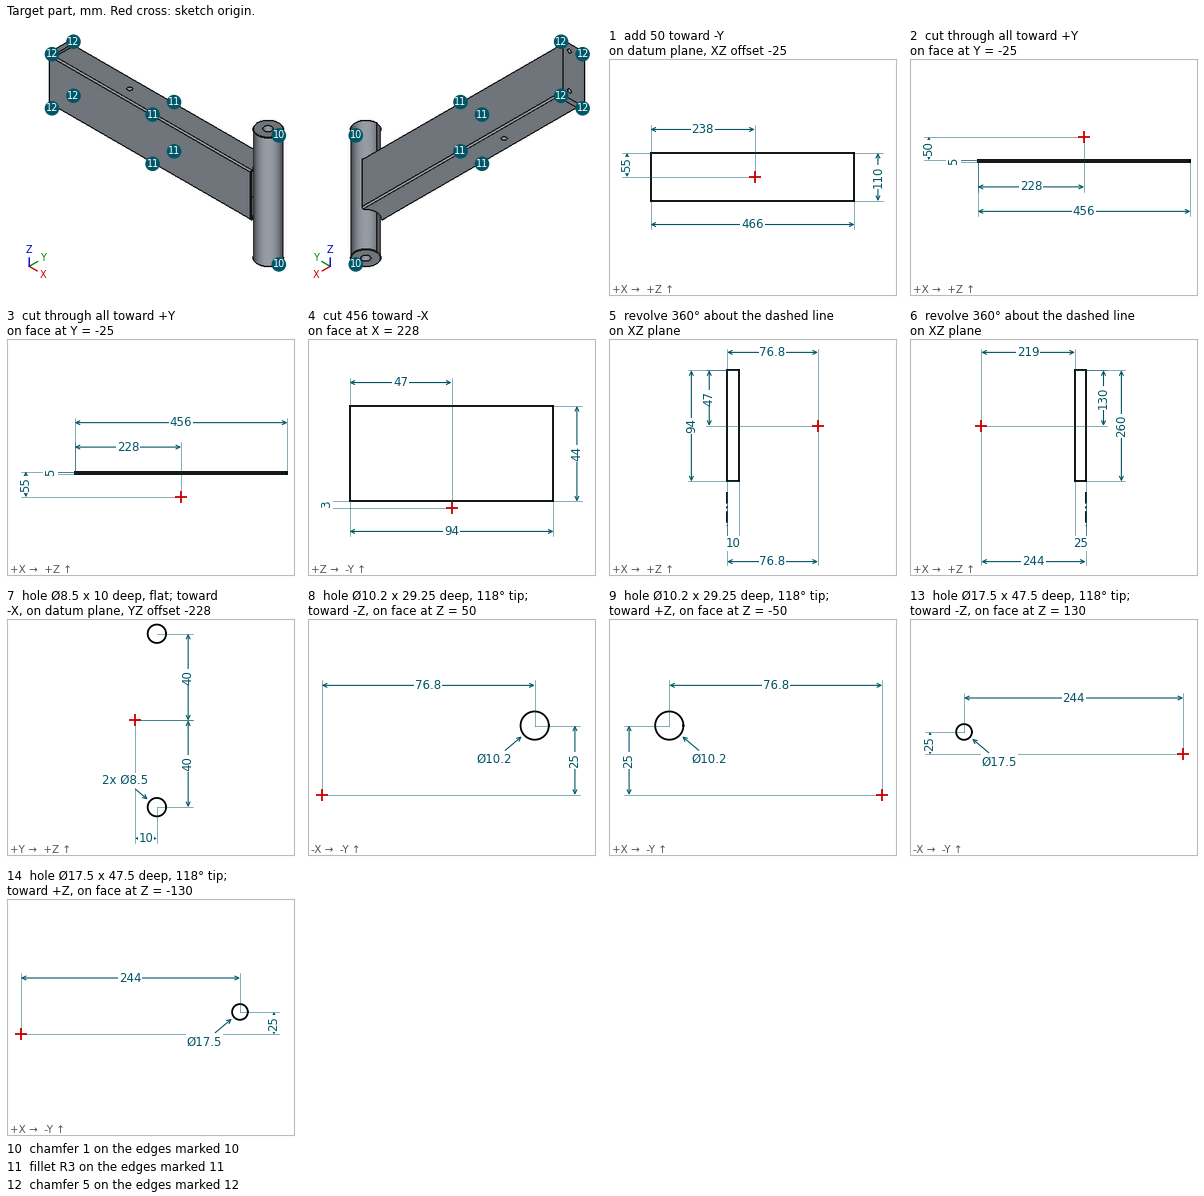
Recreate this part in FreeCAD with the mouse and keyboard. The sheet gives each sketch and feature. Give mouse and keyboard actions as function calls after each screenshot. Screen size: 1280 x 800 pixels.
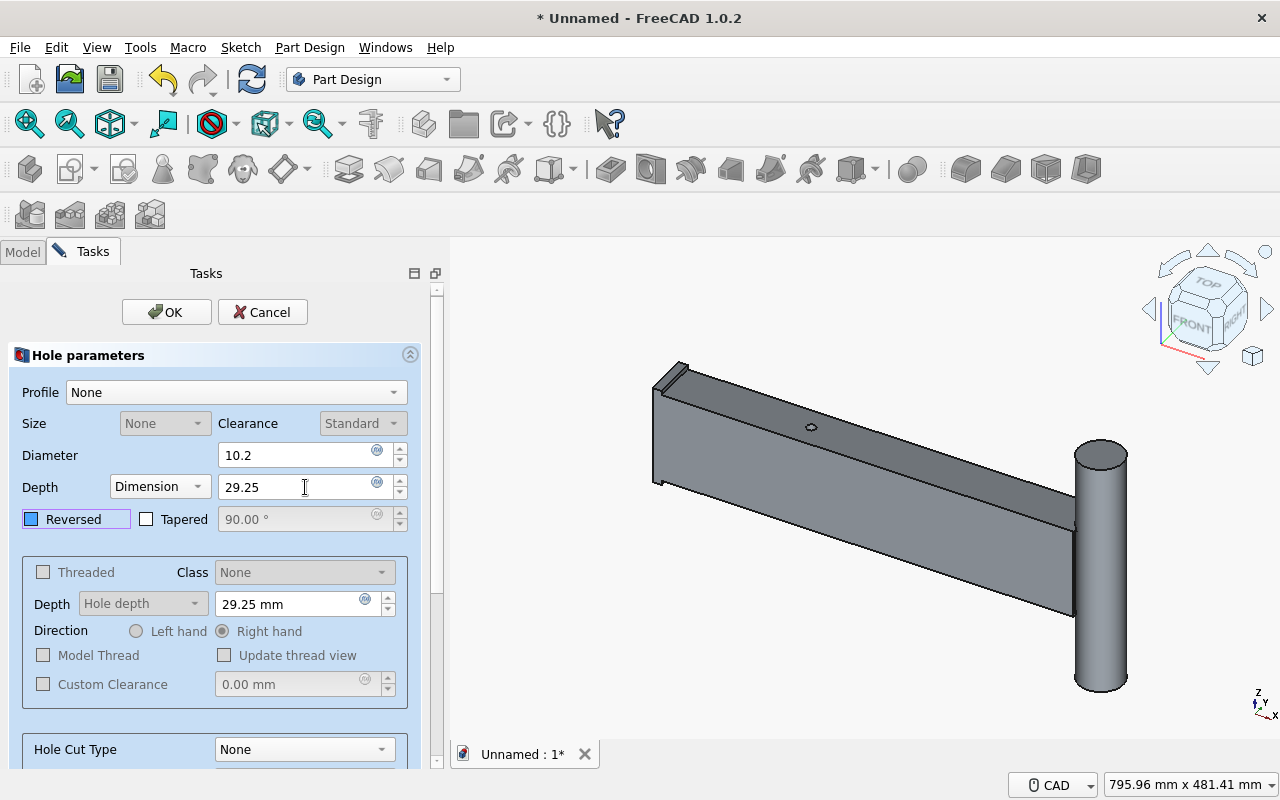
click(167, 312)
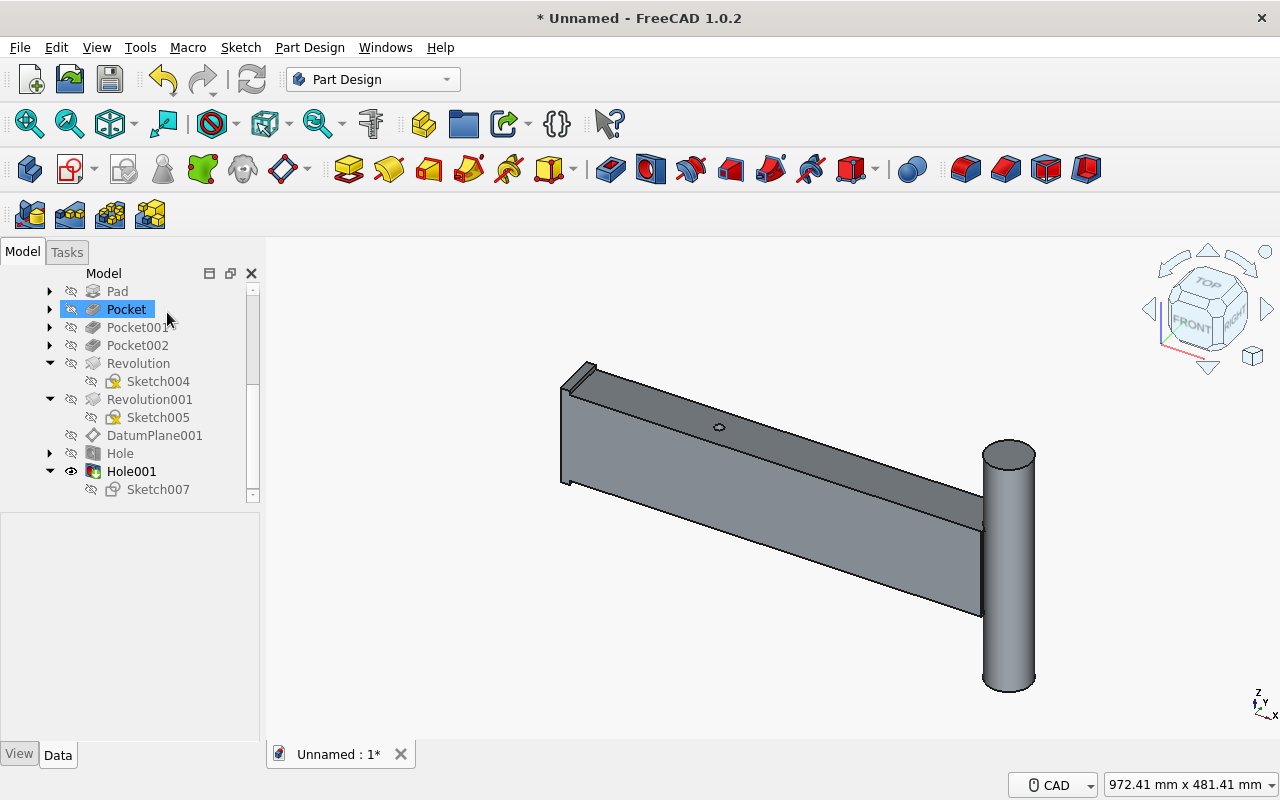
key(5)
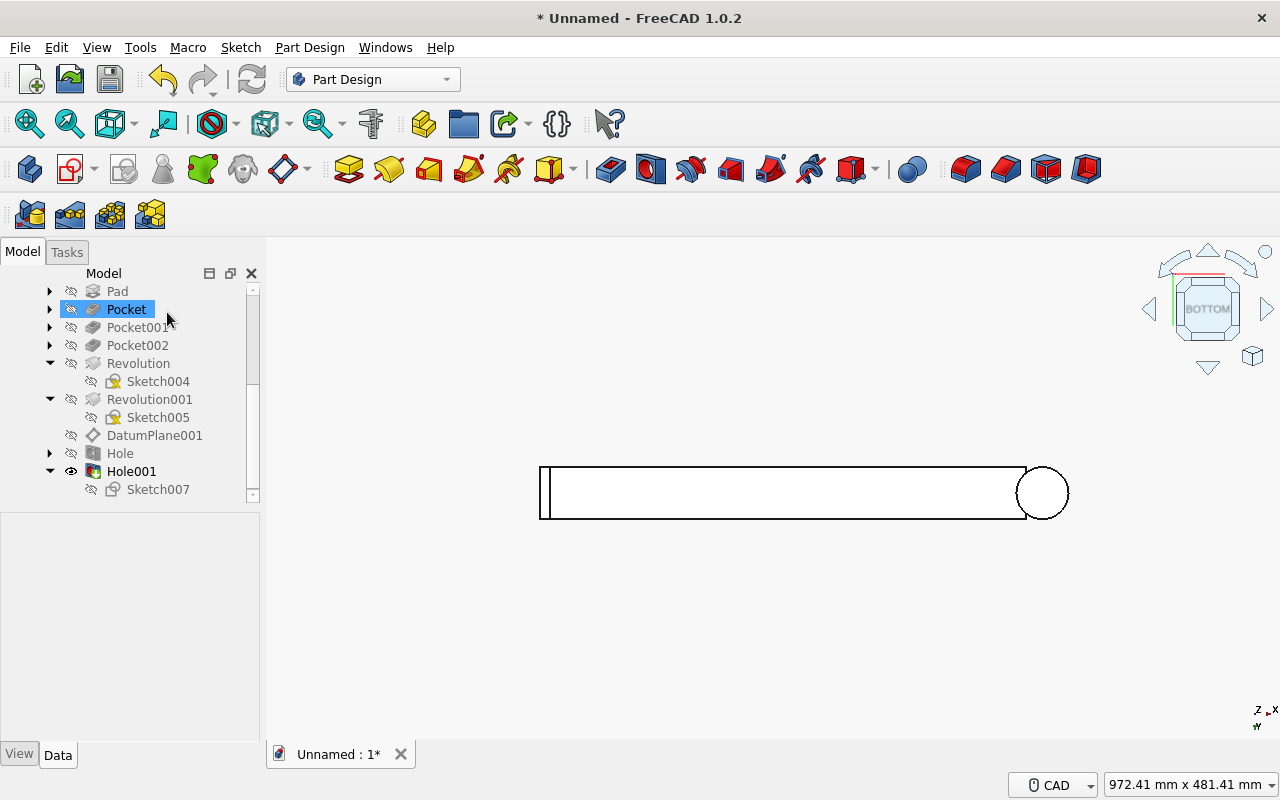
click(924, 492)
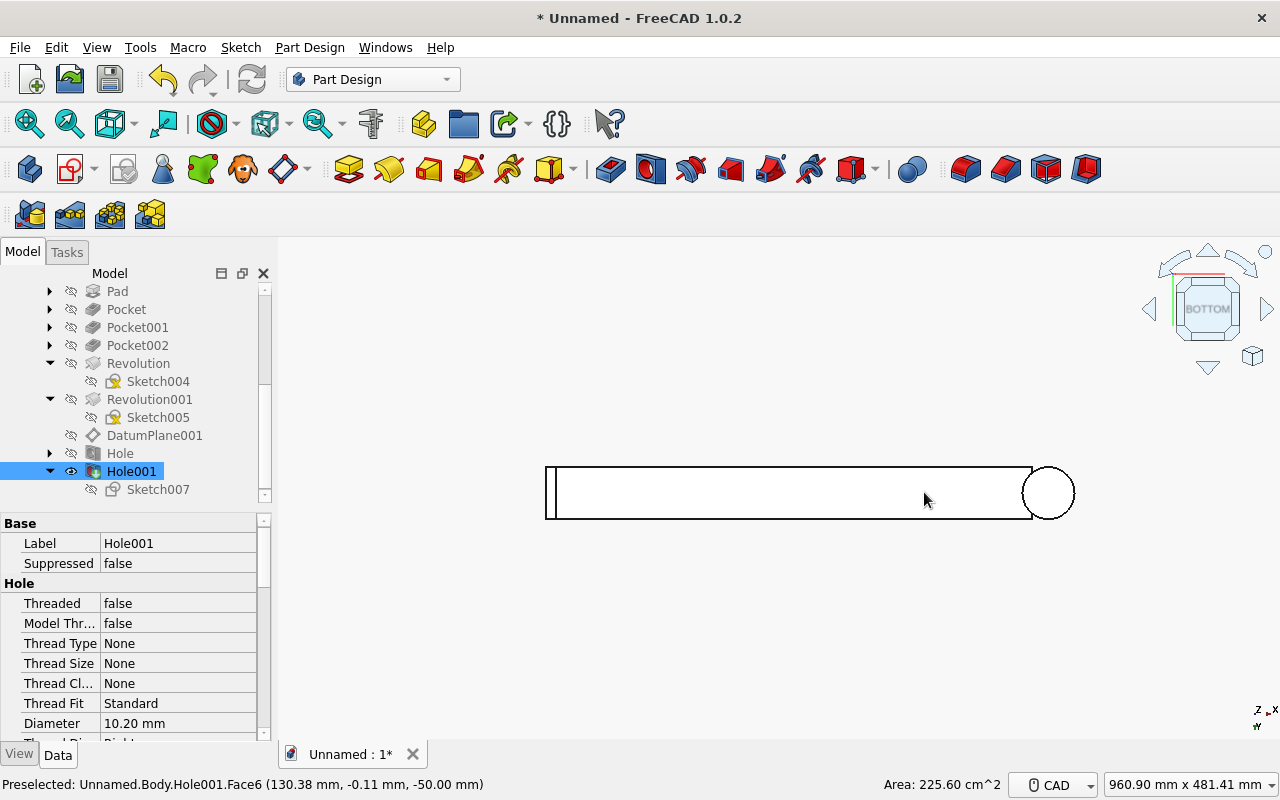
click(70, 170)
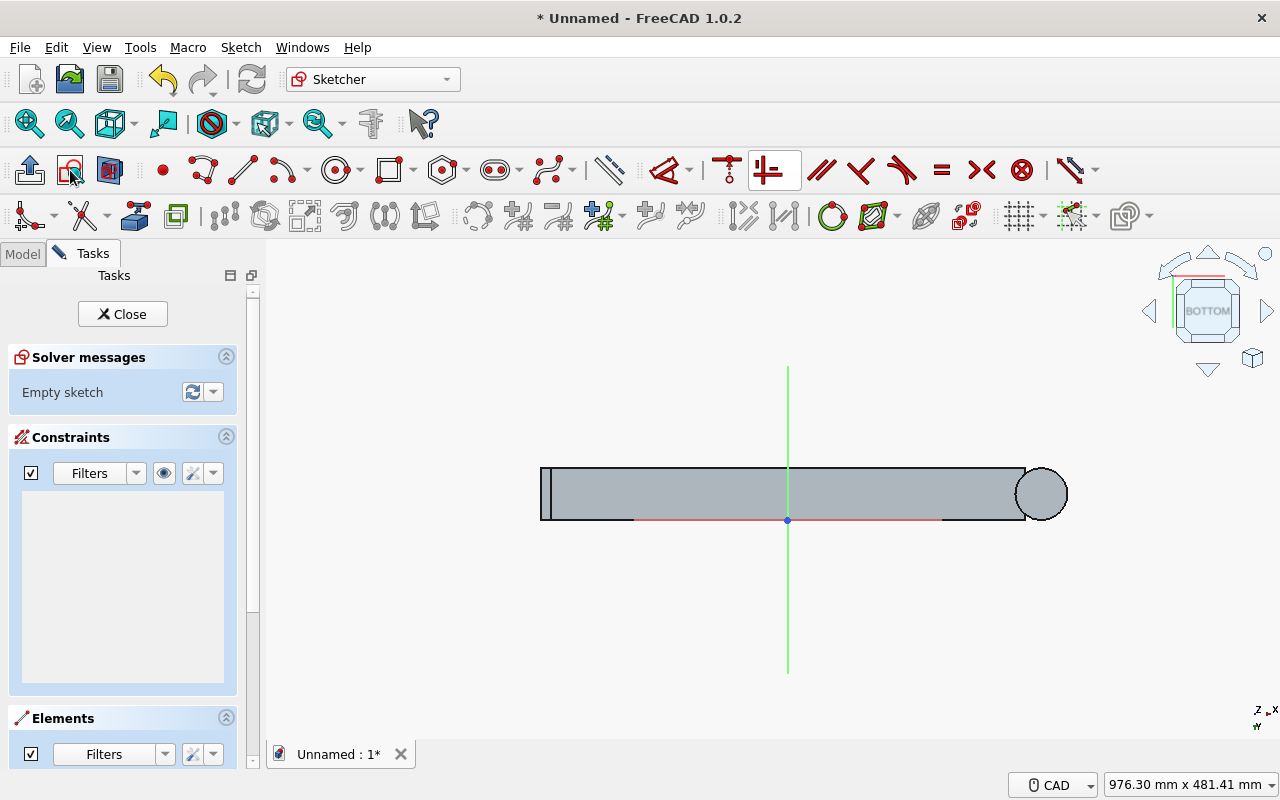
click(110, 170)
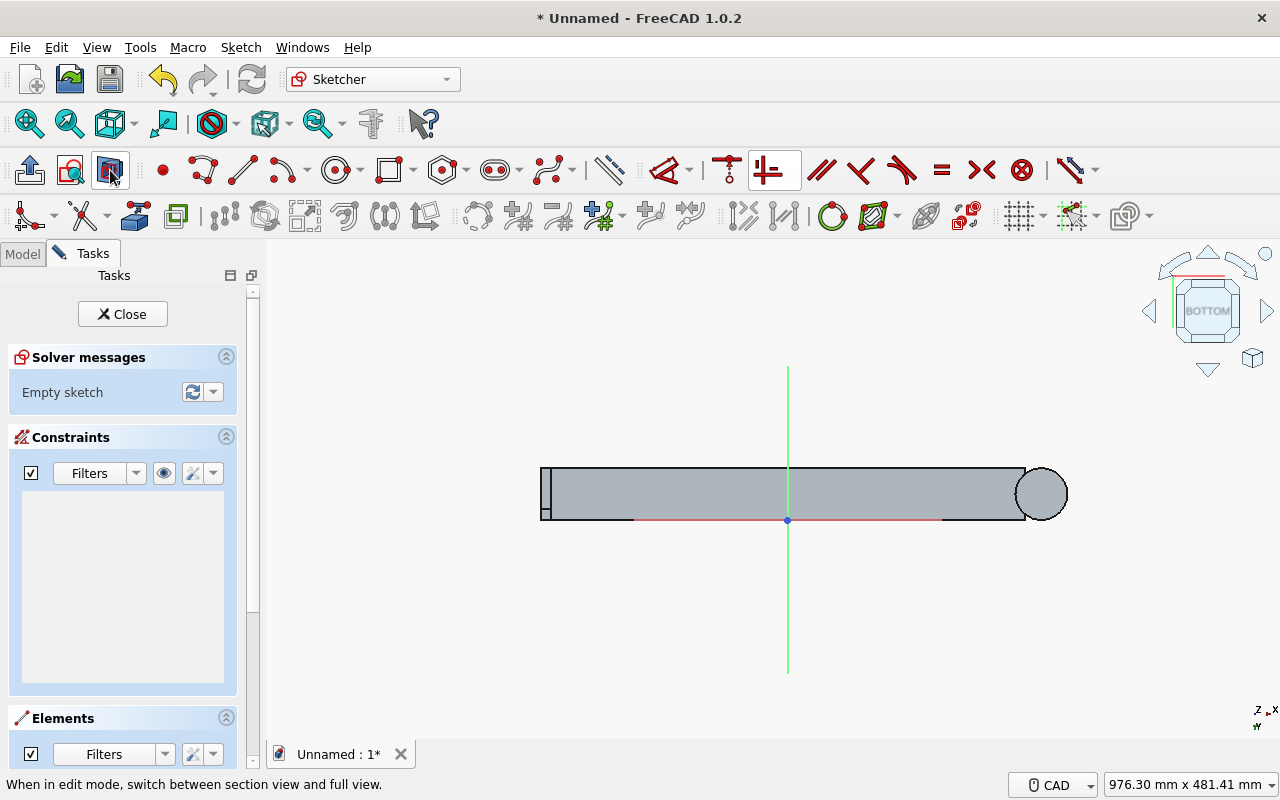
scroll(708, 494, up, 15)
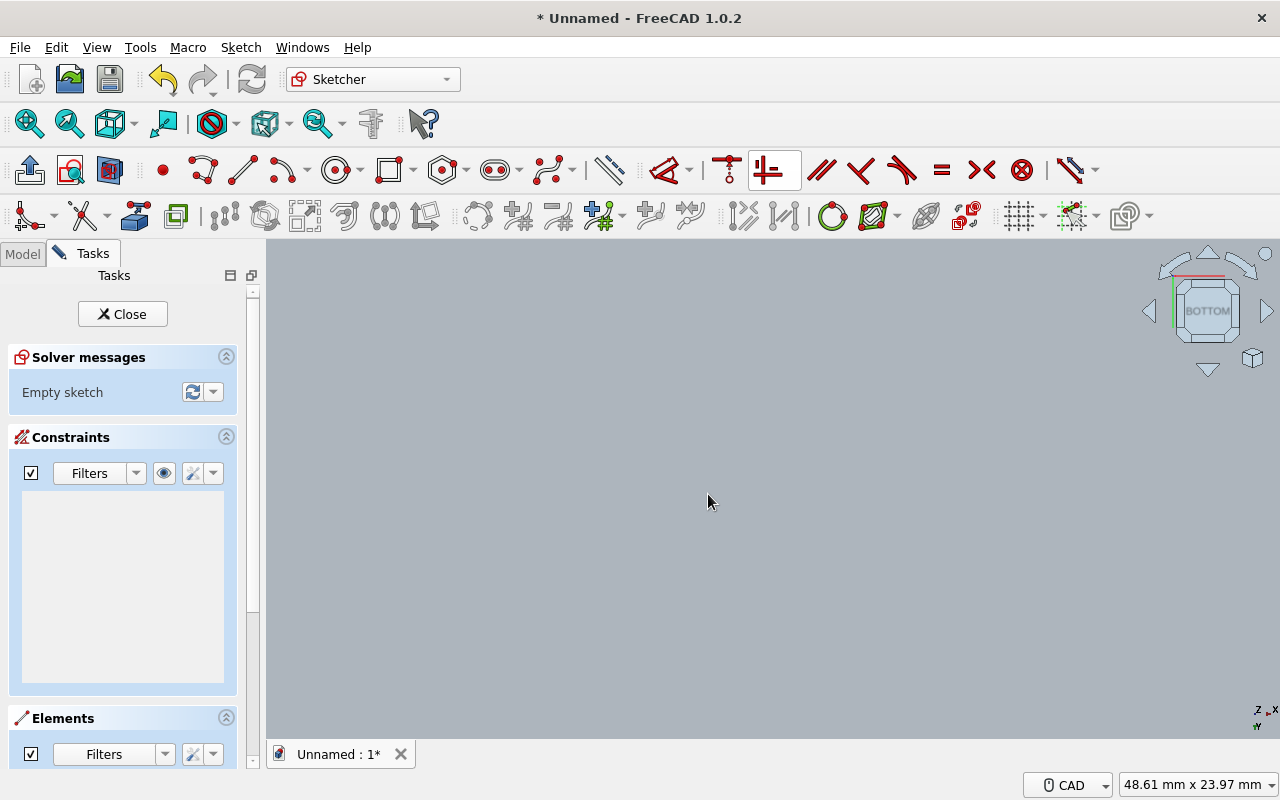
scroll(703, 481, up, 2)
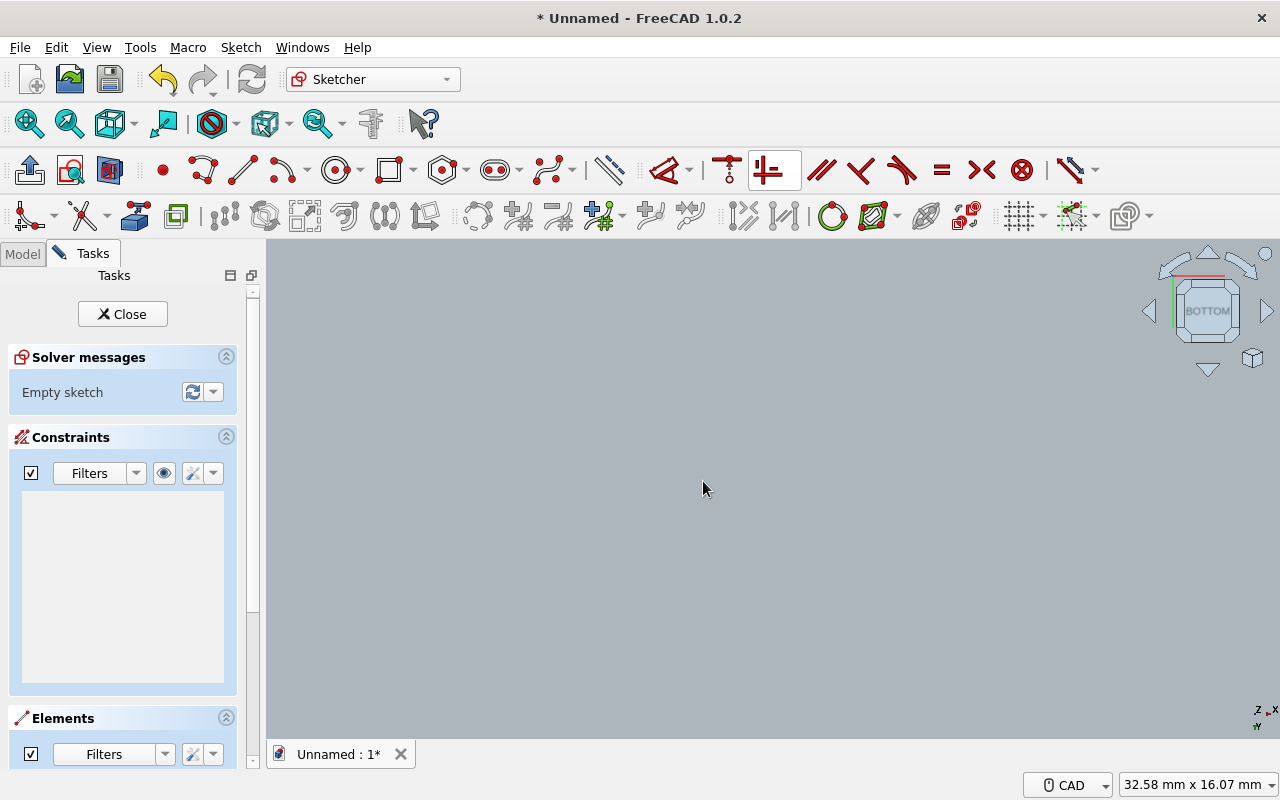
click(336, 170)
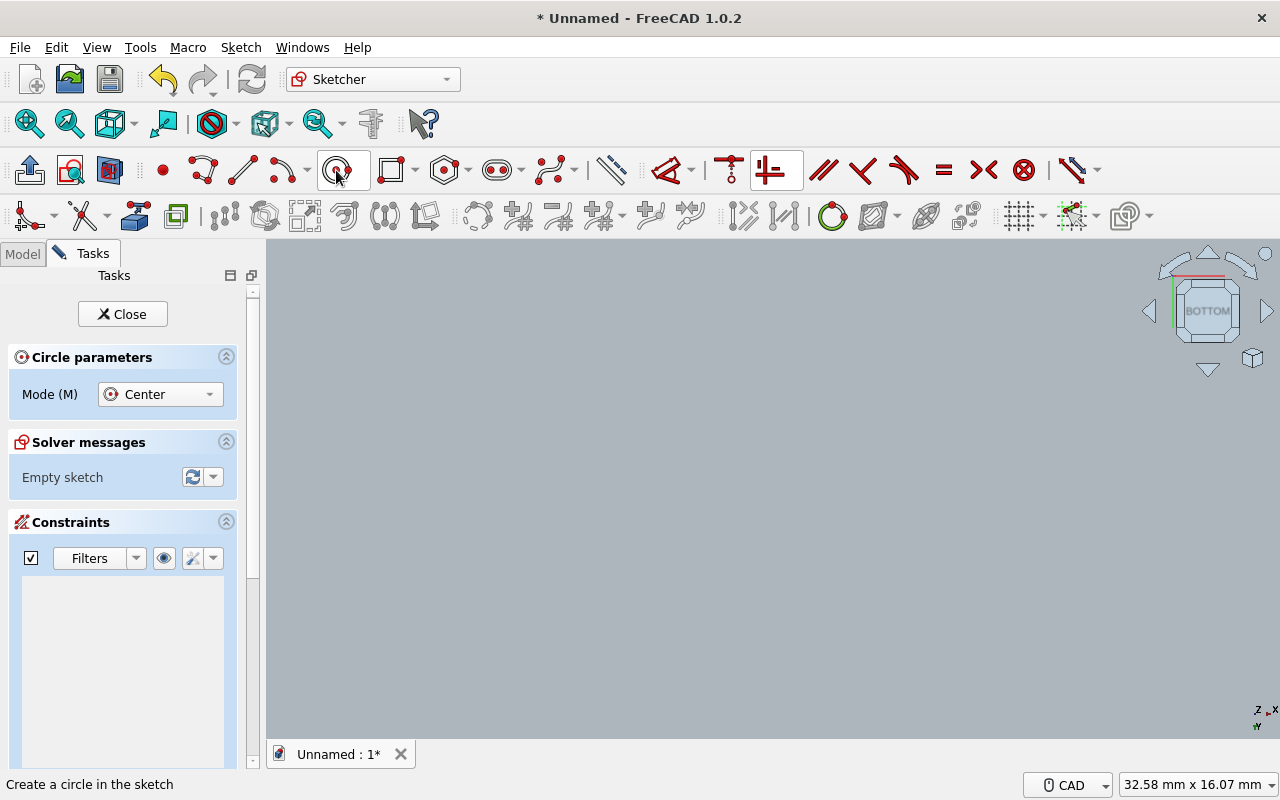
click(704, 489)
move(817, 376)